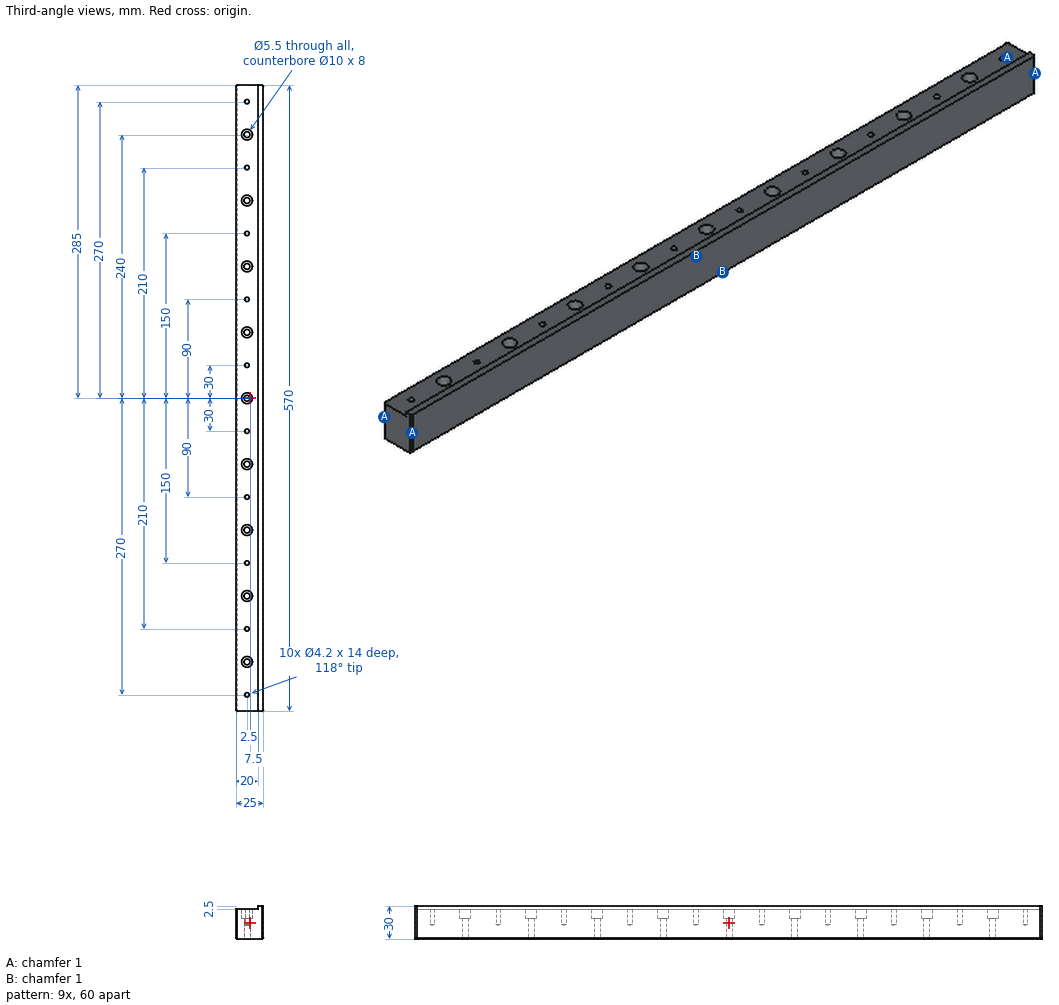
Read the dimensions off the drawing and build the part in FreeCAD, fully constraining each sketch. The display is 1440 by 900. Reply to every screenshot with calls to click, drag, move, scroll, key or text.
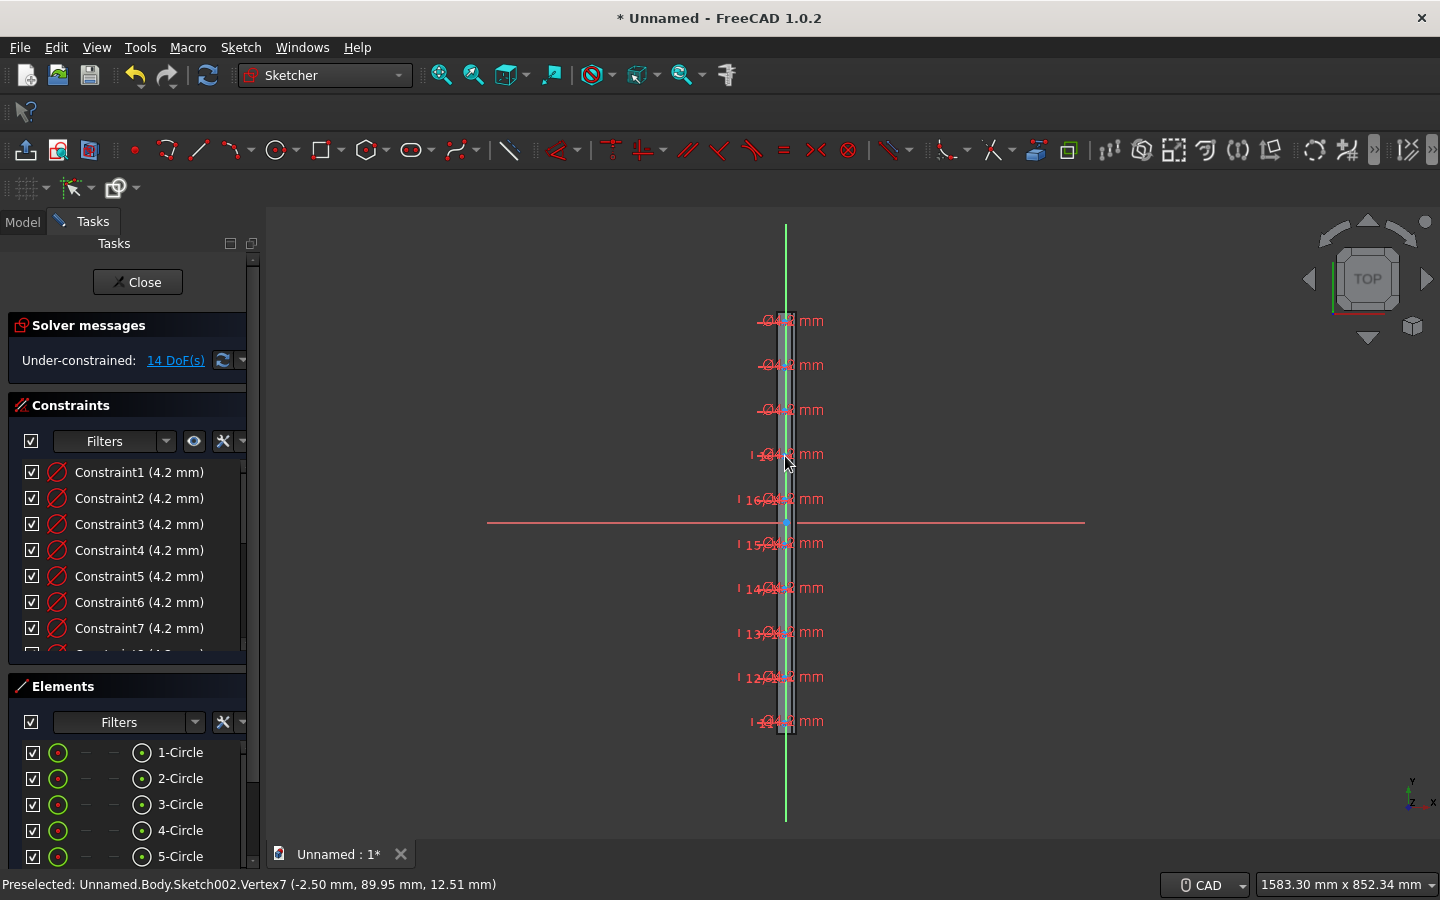
click(785, 456)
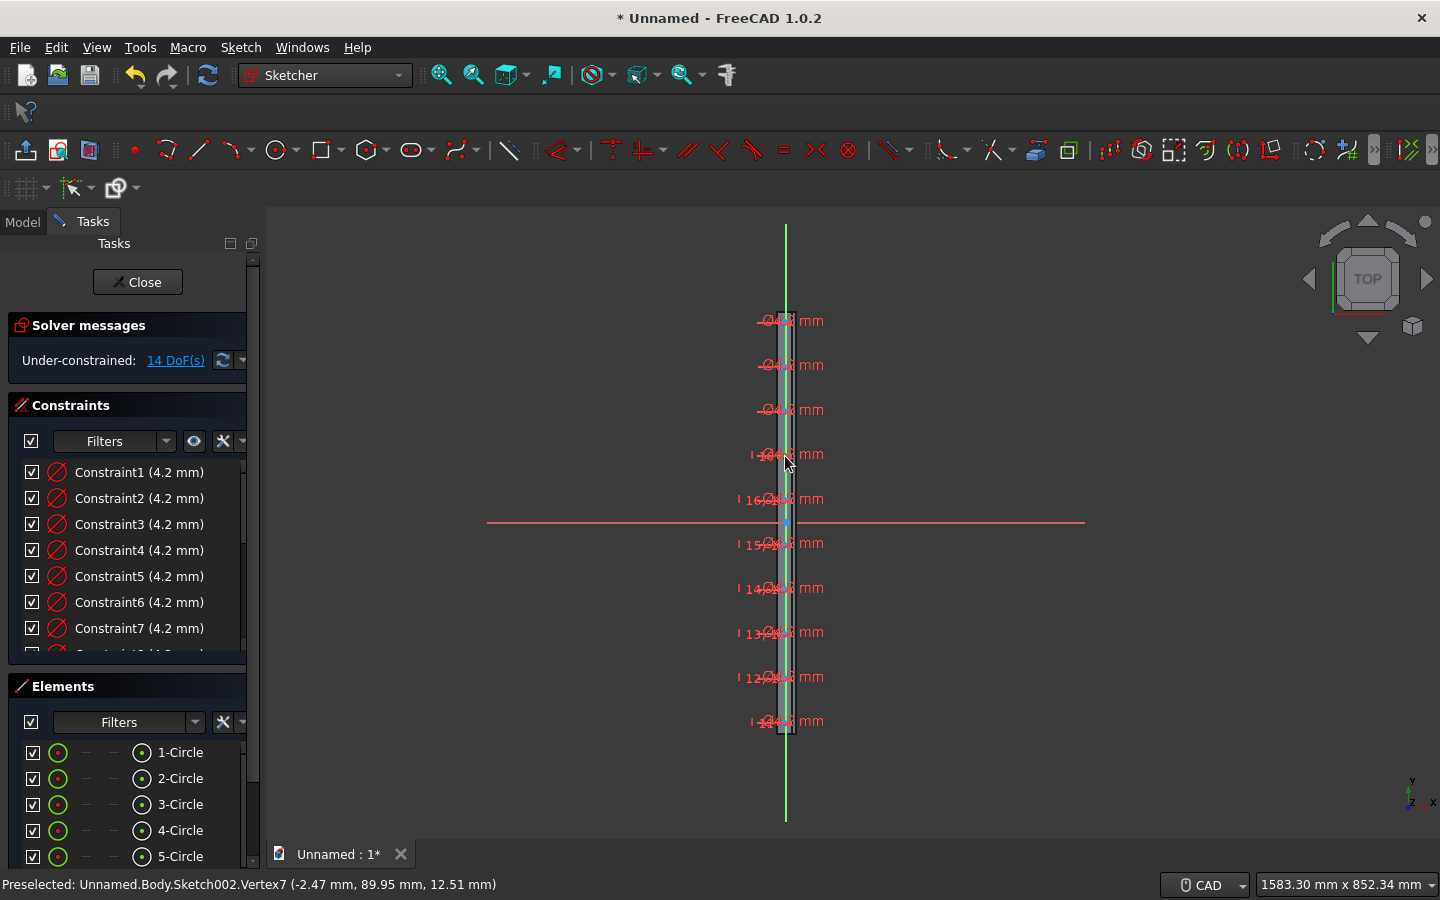
click(785, 412)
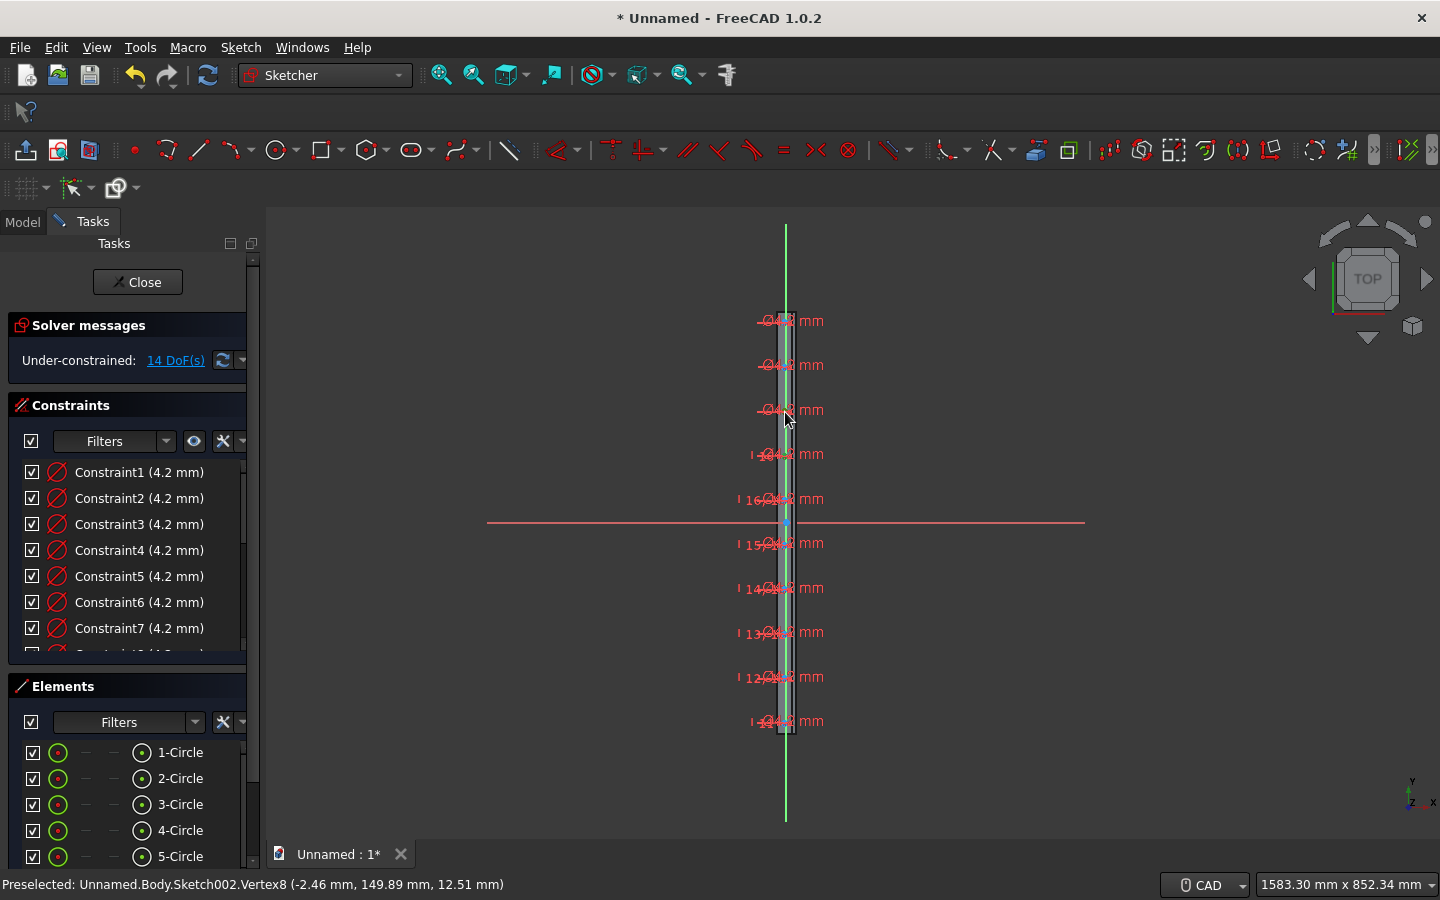
click(666, 150)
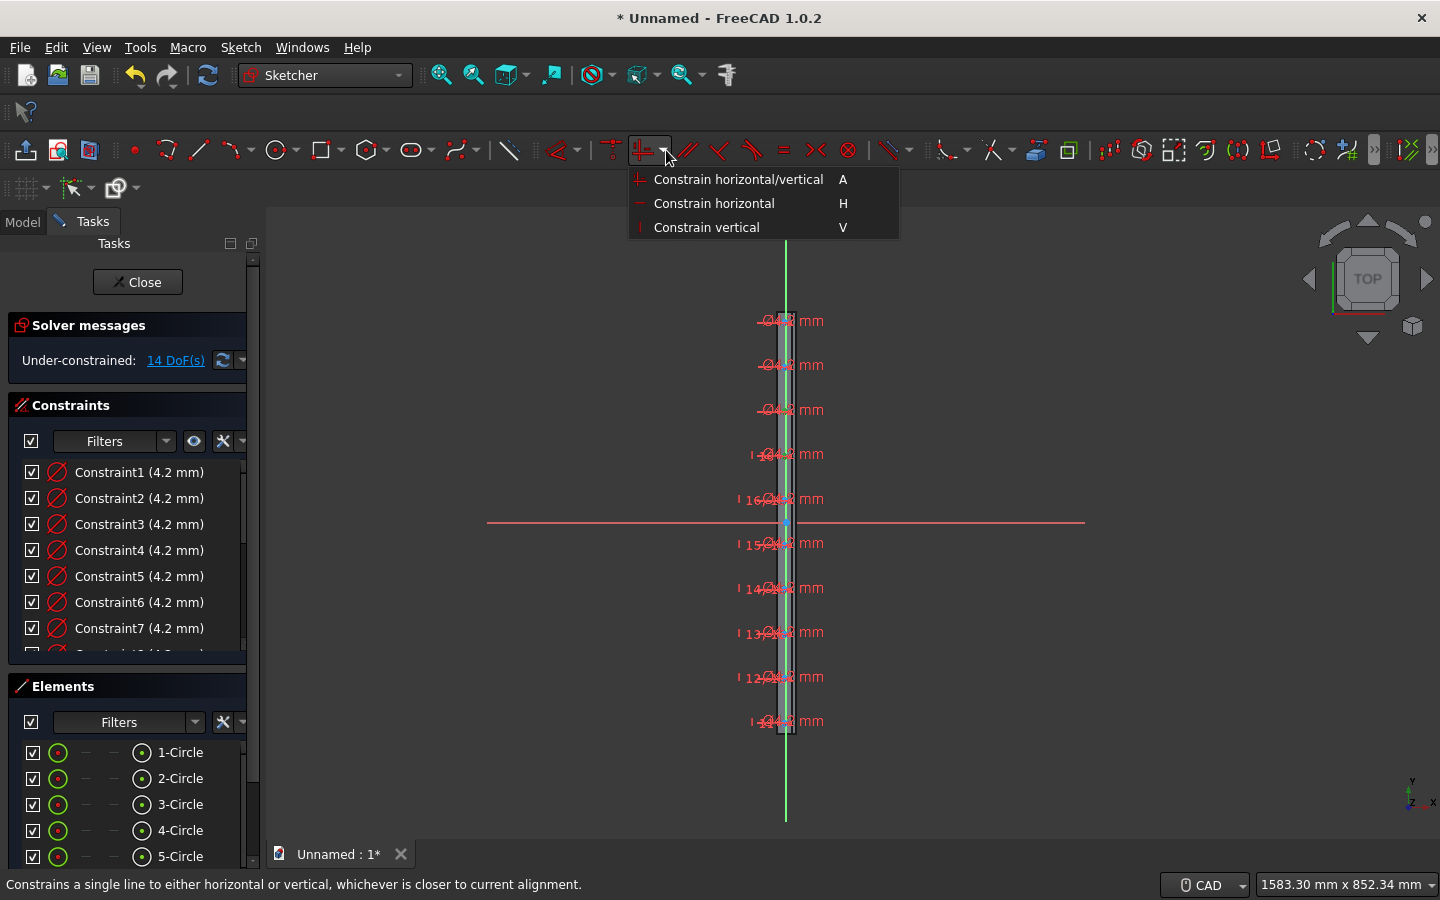
click(764, 227)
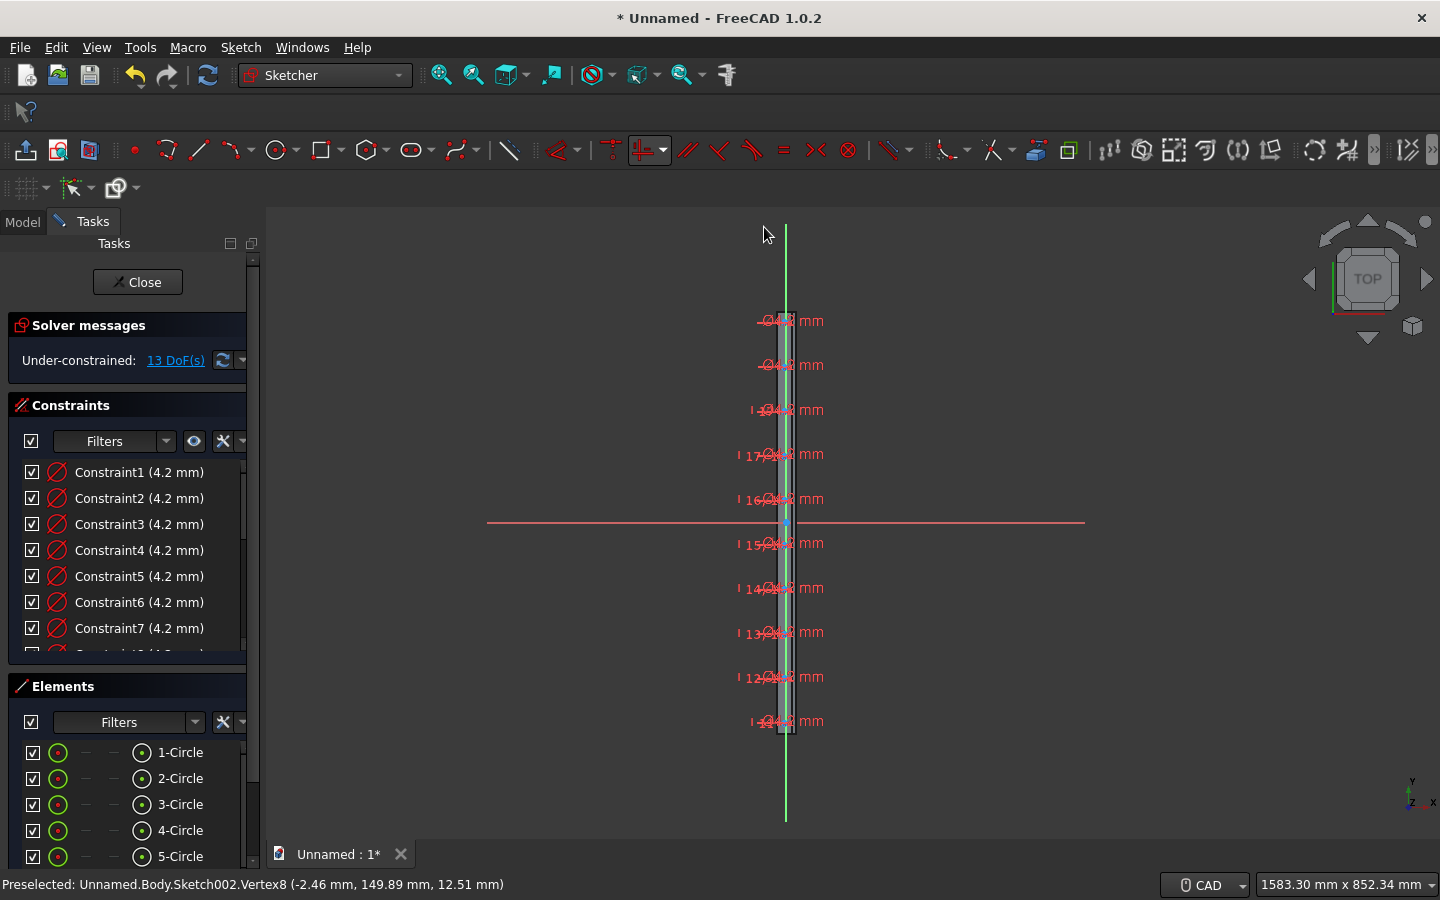
click(785, 412)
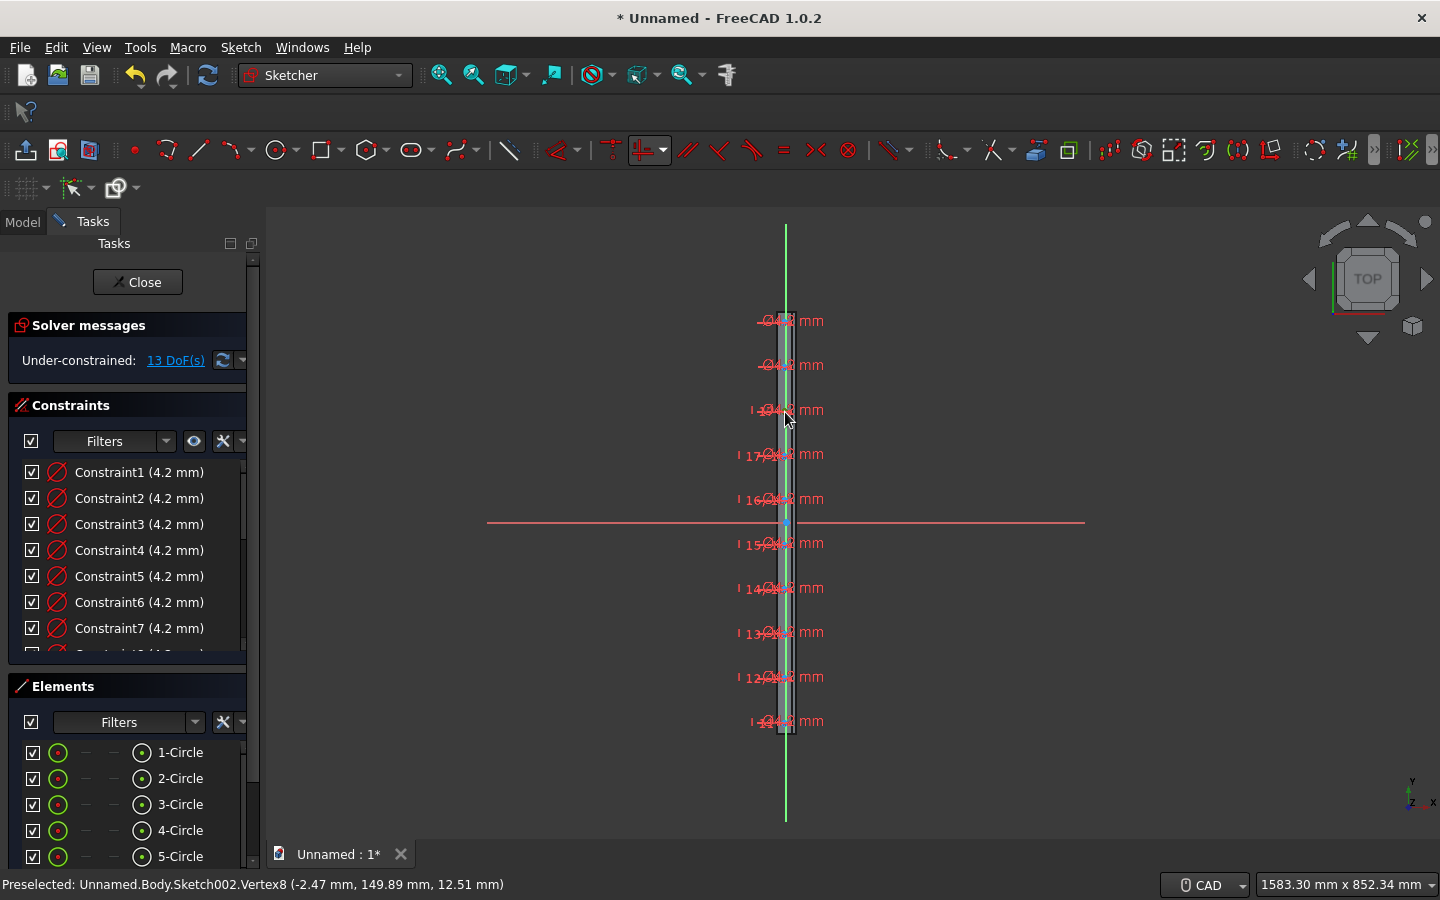
click(785, 367)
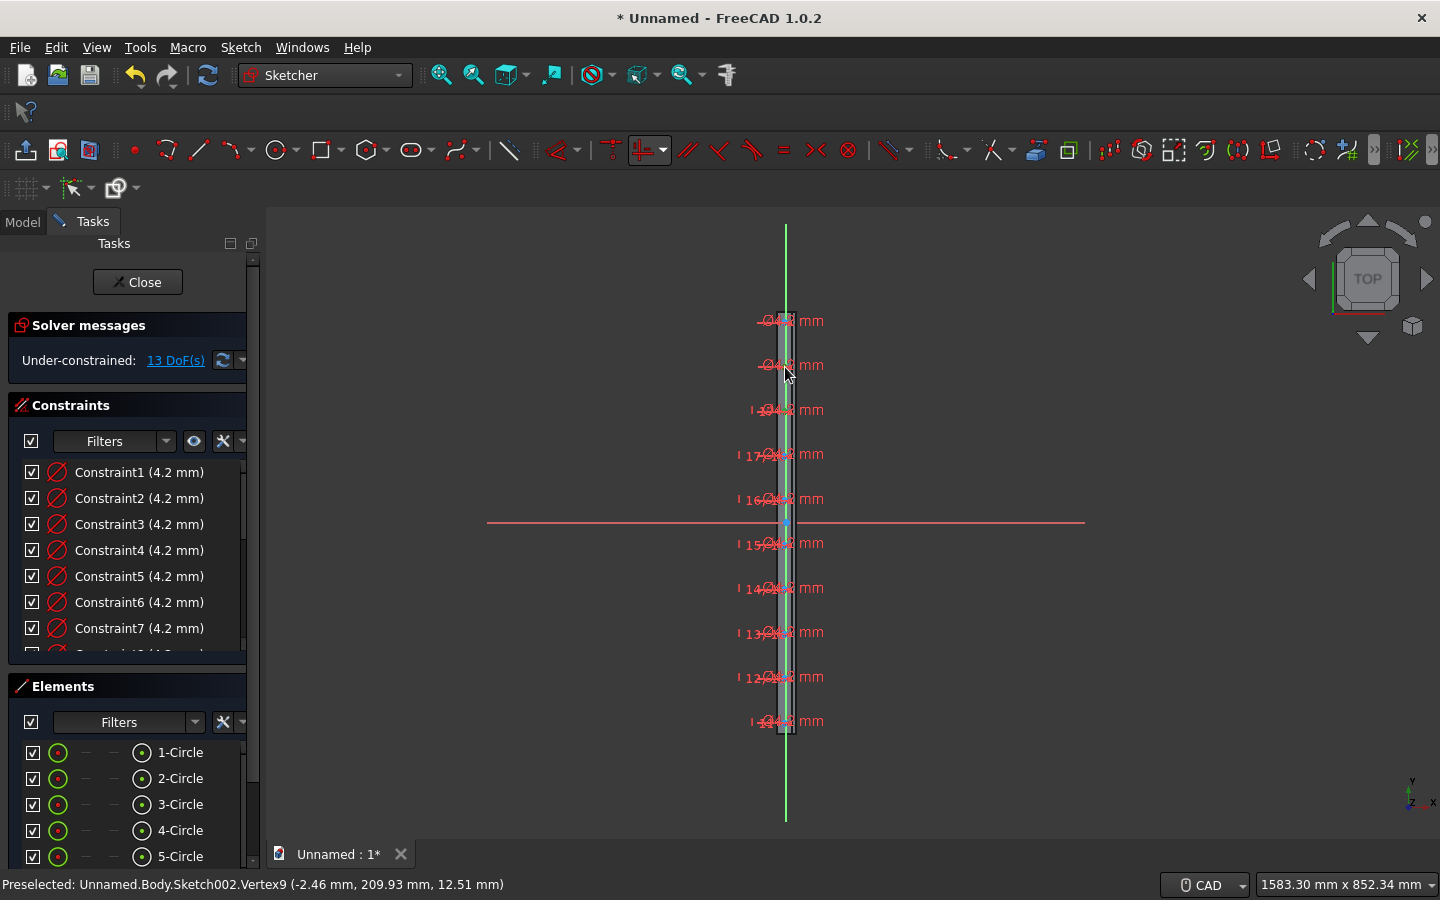
click(666, 150)